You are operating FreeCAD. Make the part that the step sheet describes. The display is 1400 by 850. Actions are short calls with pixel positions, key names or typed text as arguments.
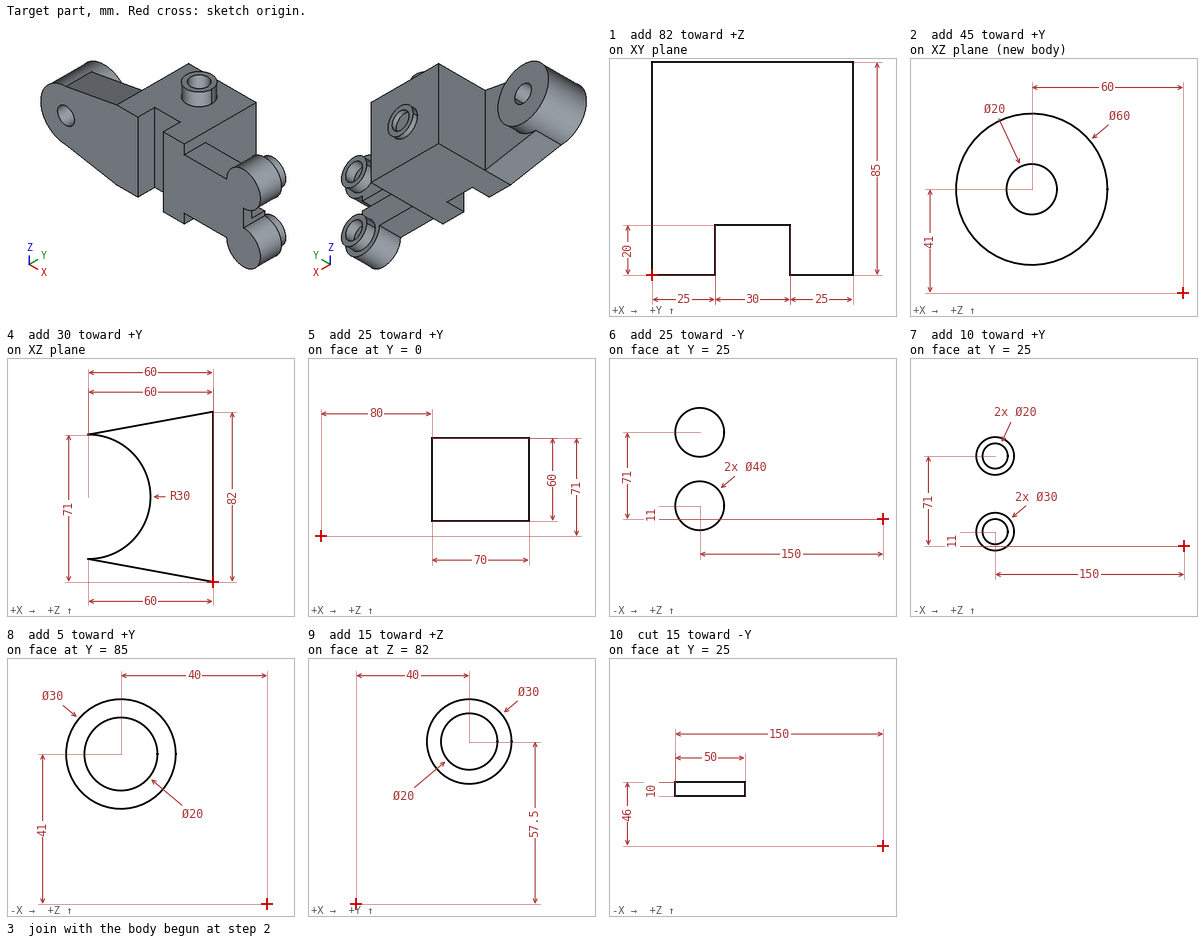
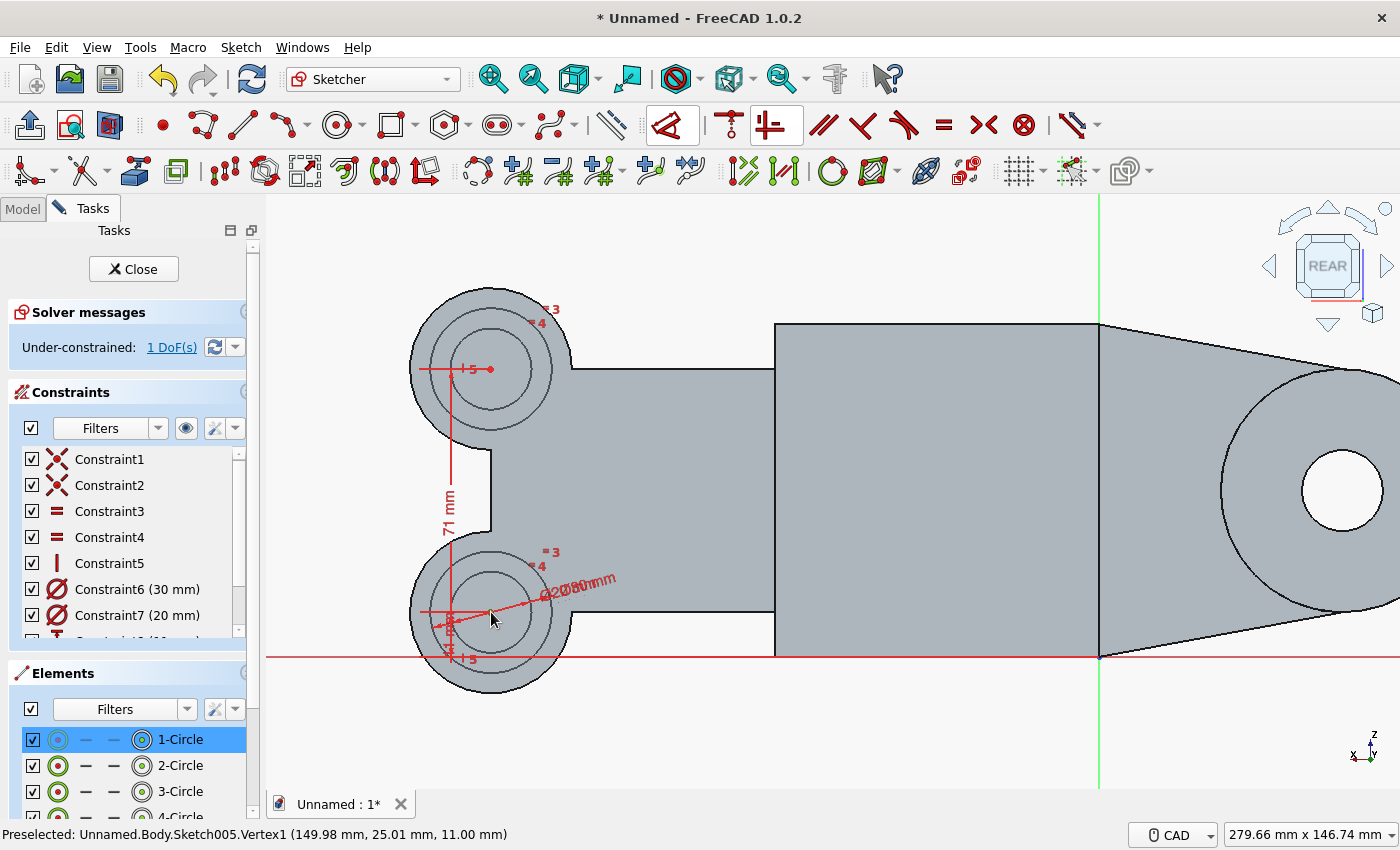
click(694, 126)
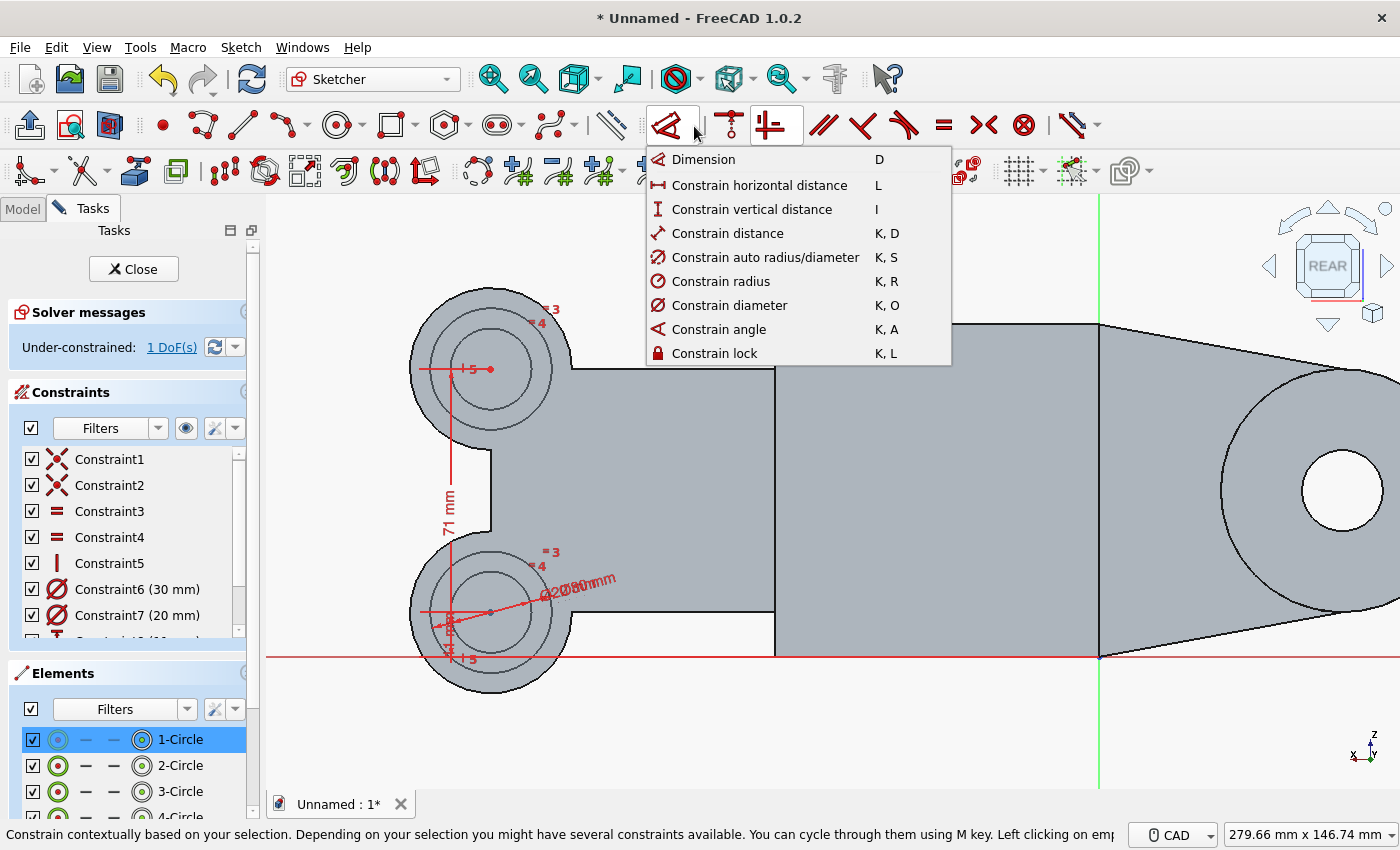
click(799, 185)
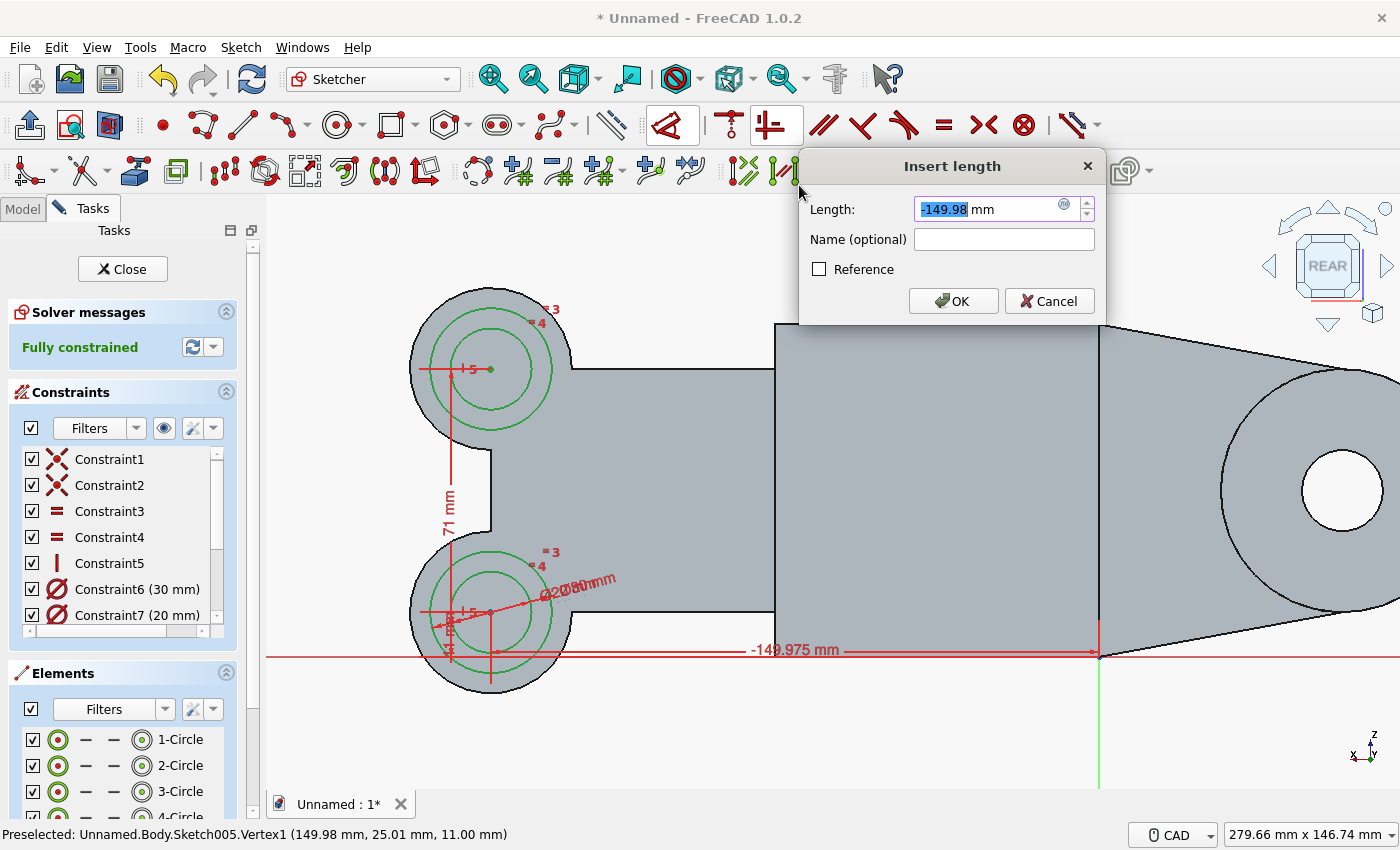
text(-150)
key(Return)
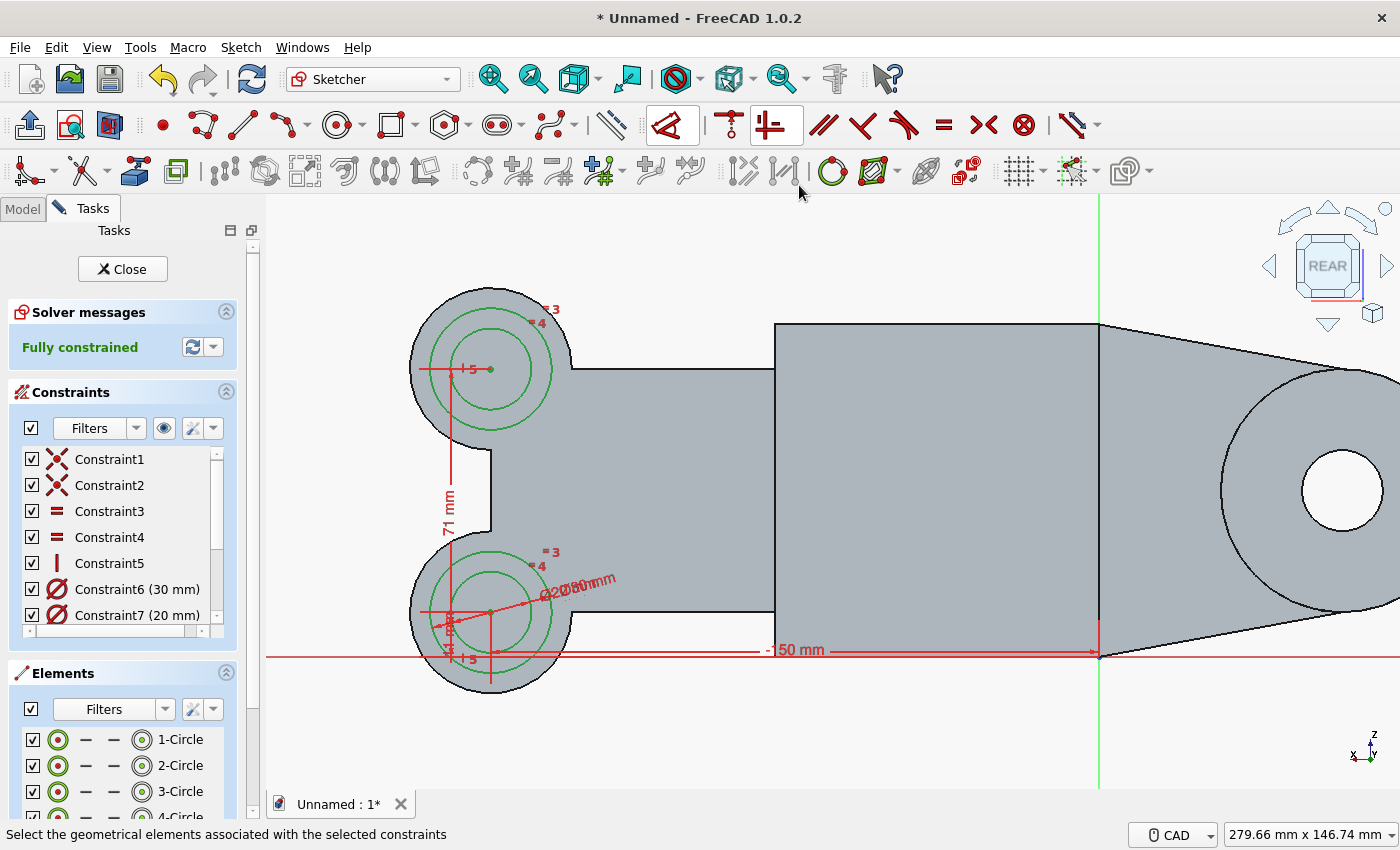
click(123, 269)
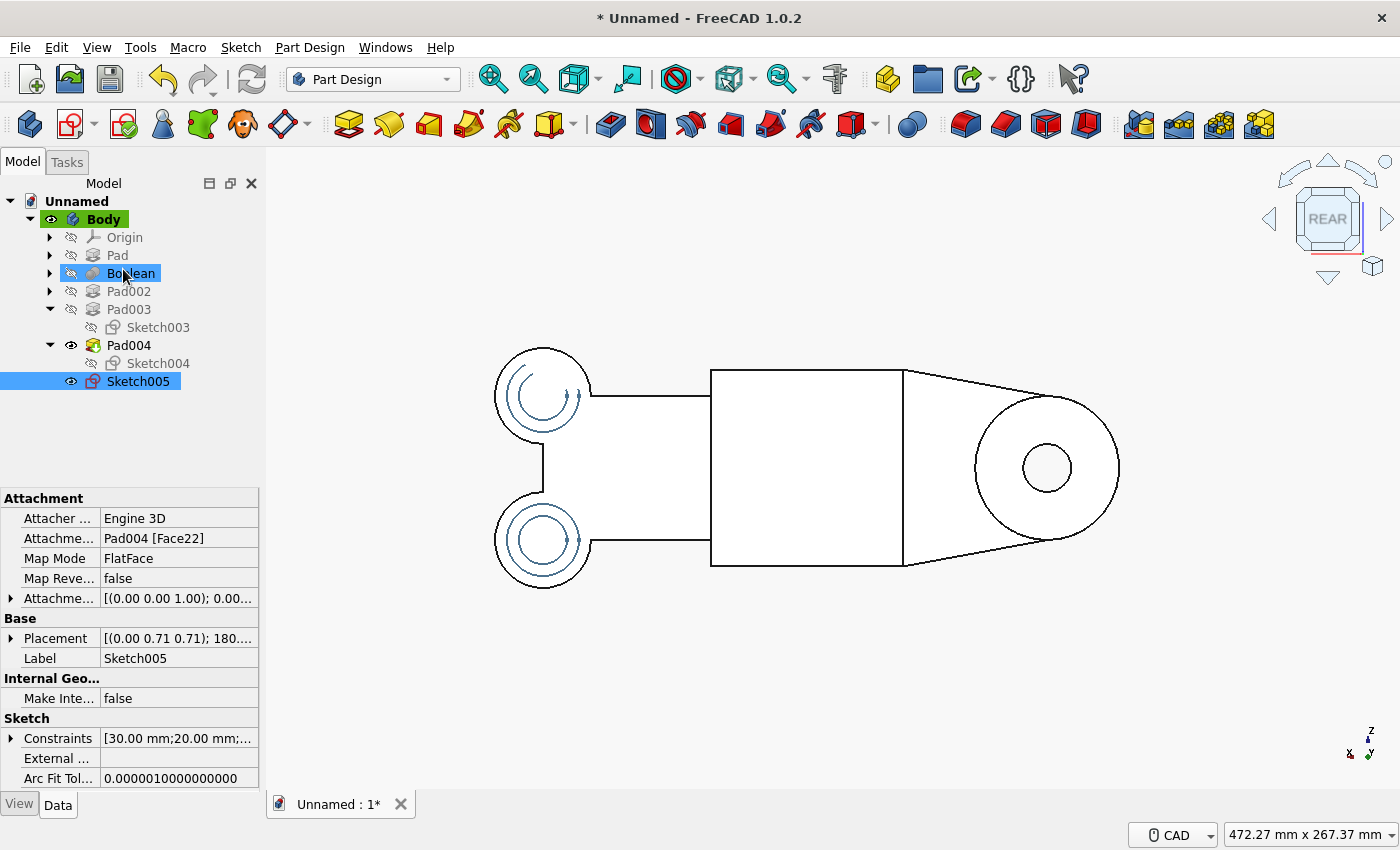
click(350, 124)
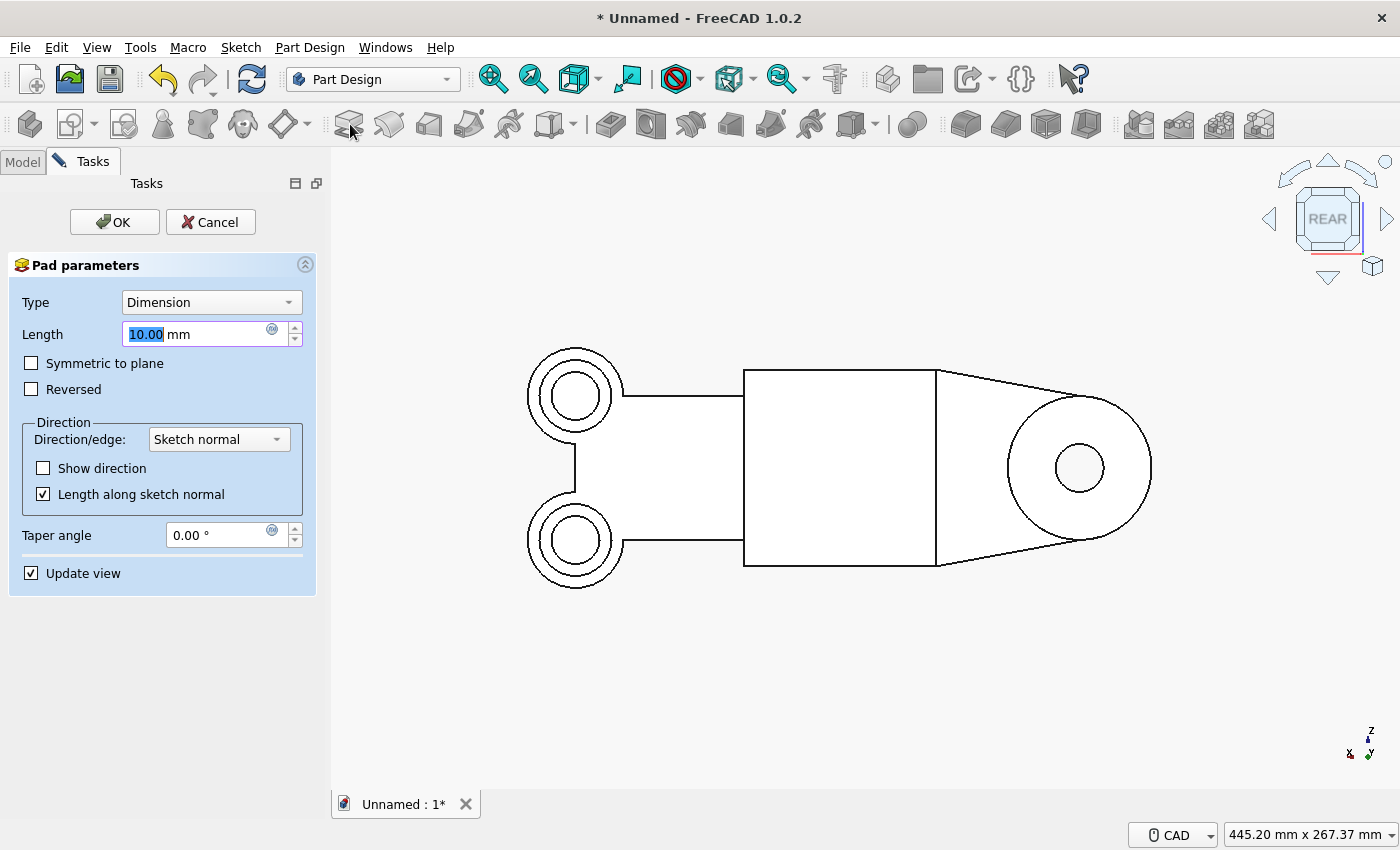
text(10)
key(Tab)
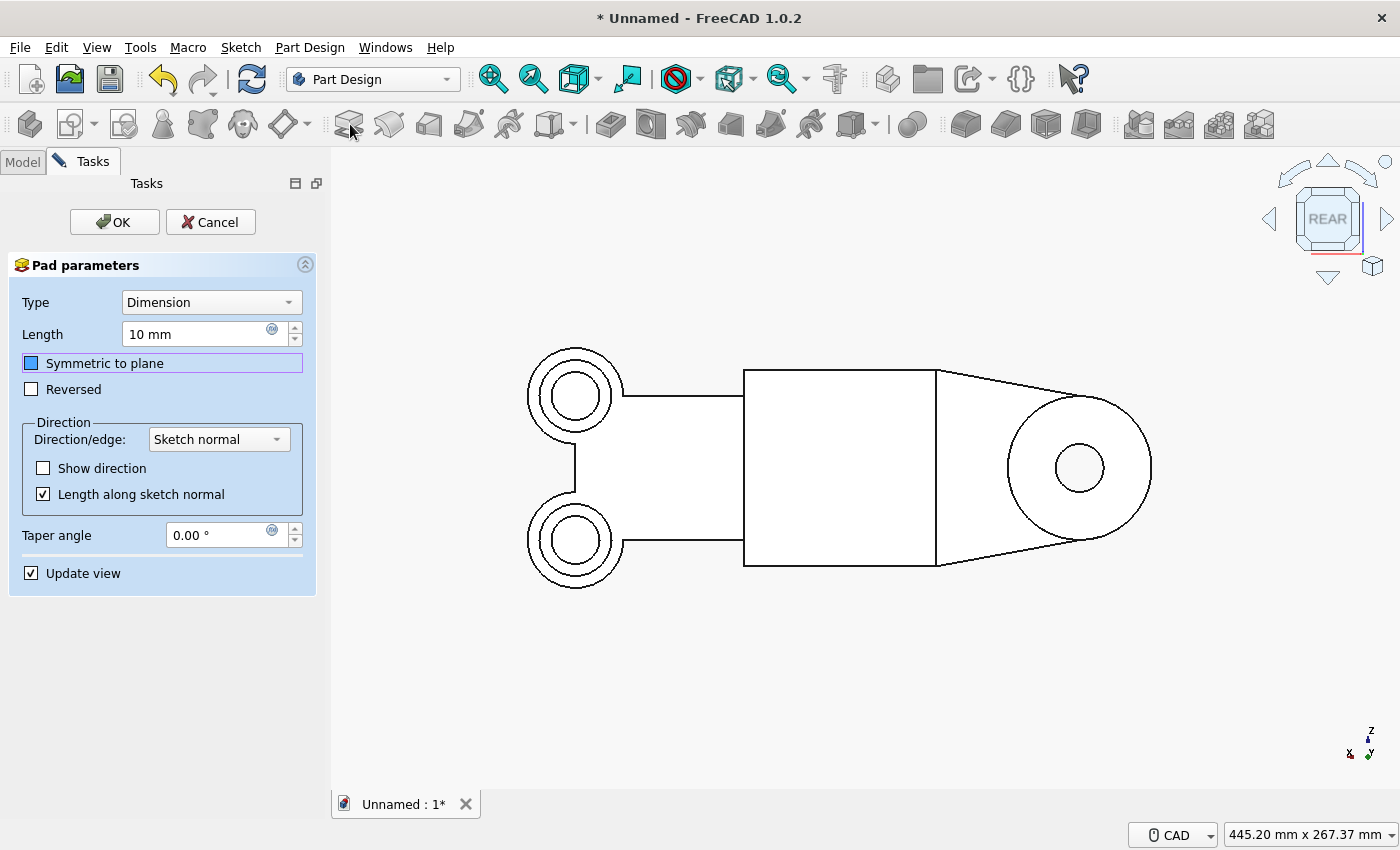
click(115, 222)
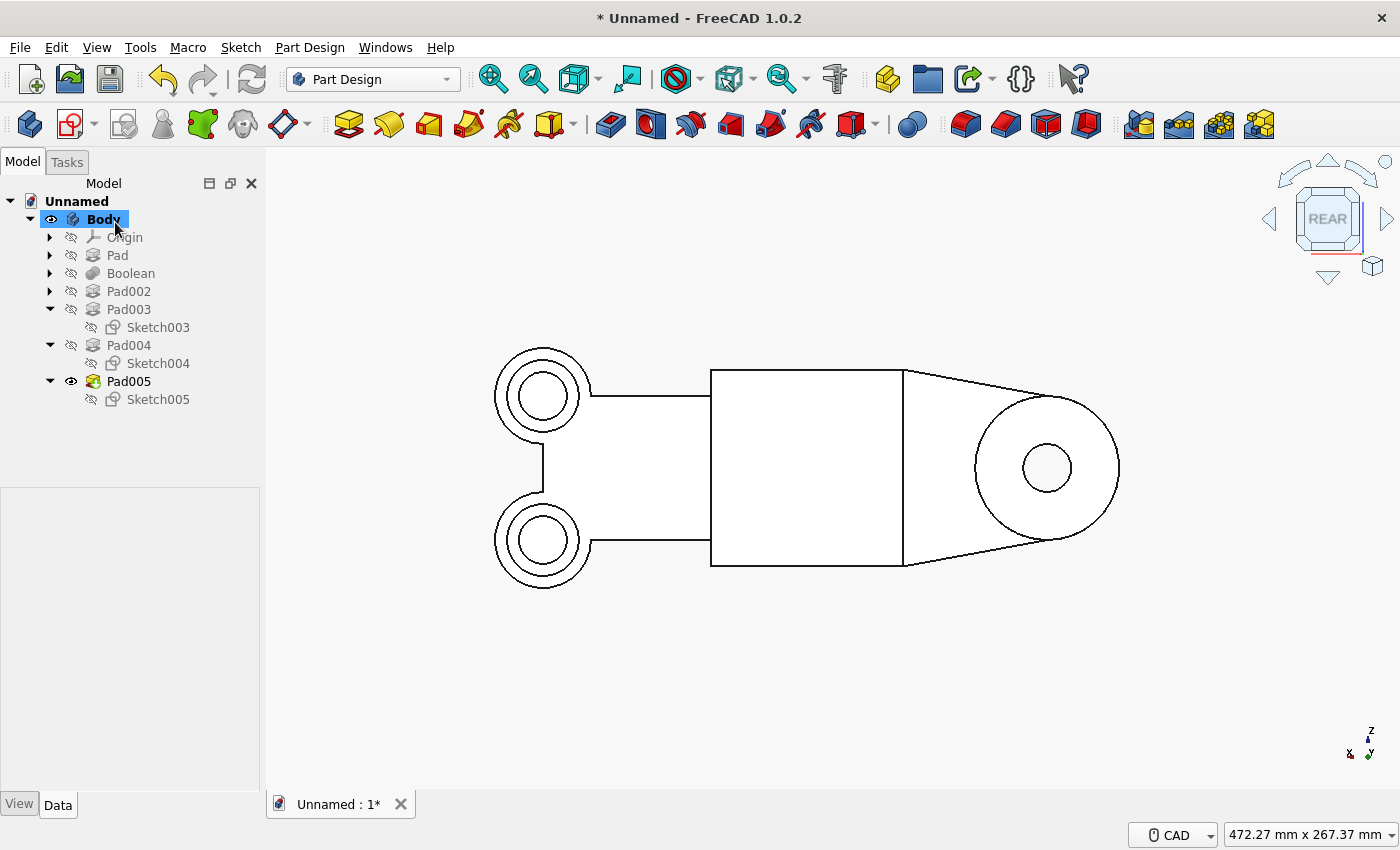
click(807, 467)